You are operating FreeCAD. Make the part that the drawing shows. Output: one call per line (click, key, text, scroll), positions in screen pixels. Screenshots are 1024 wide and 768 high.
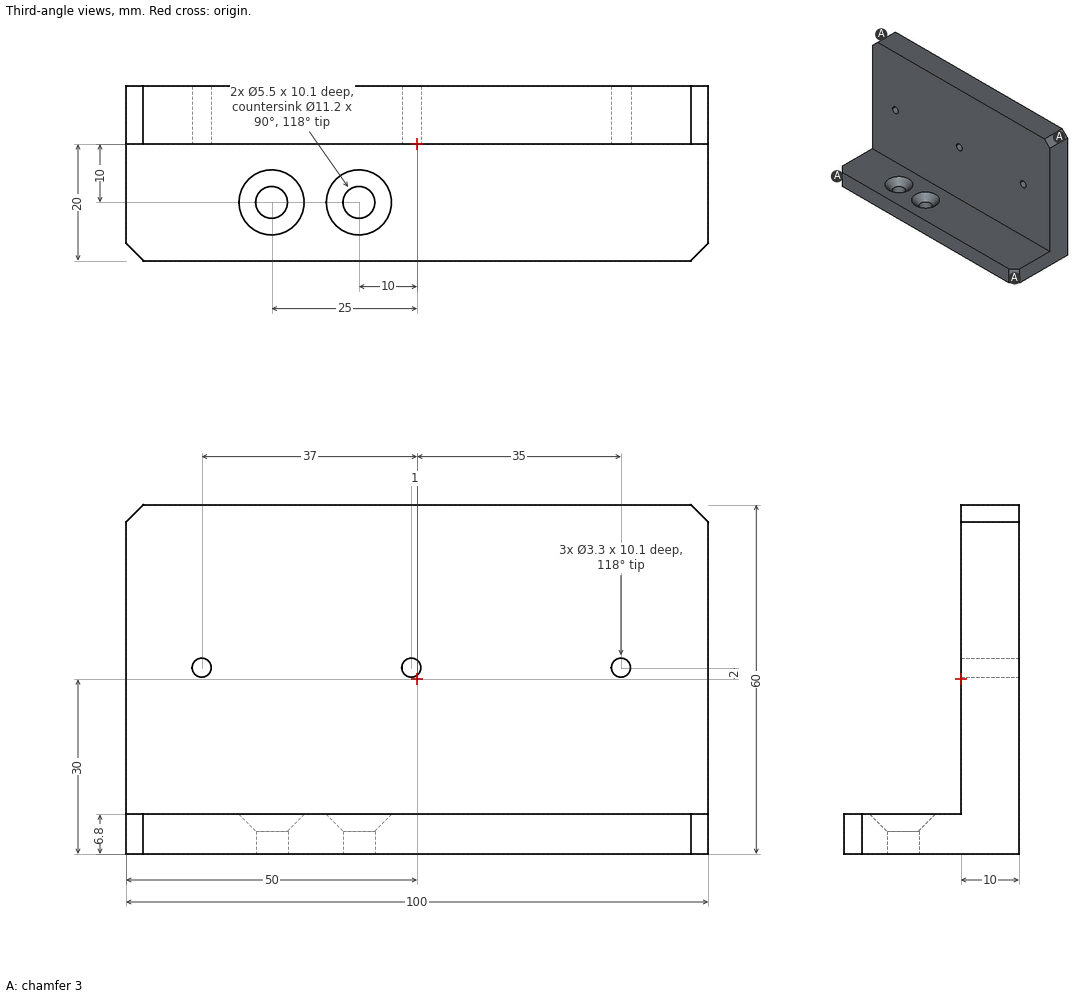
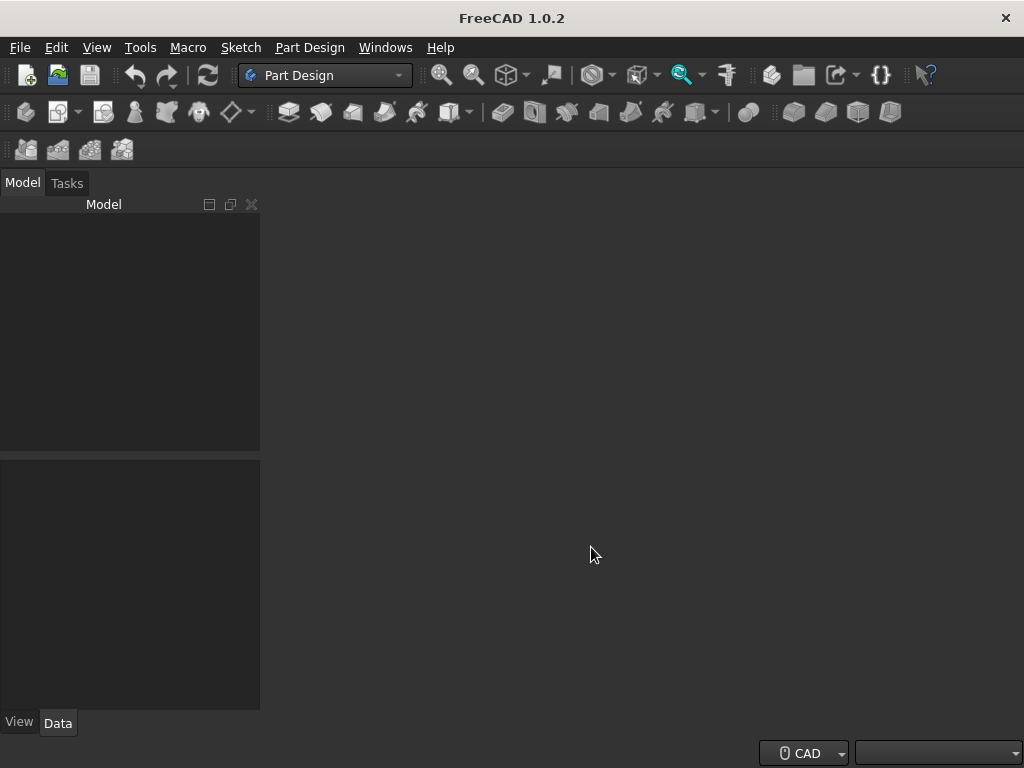
click(26, 76)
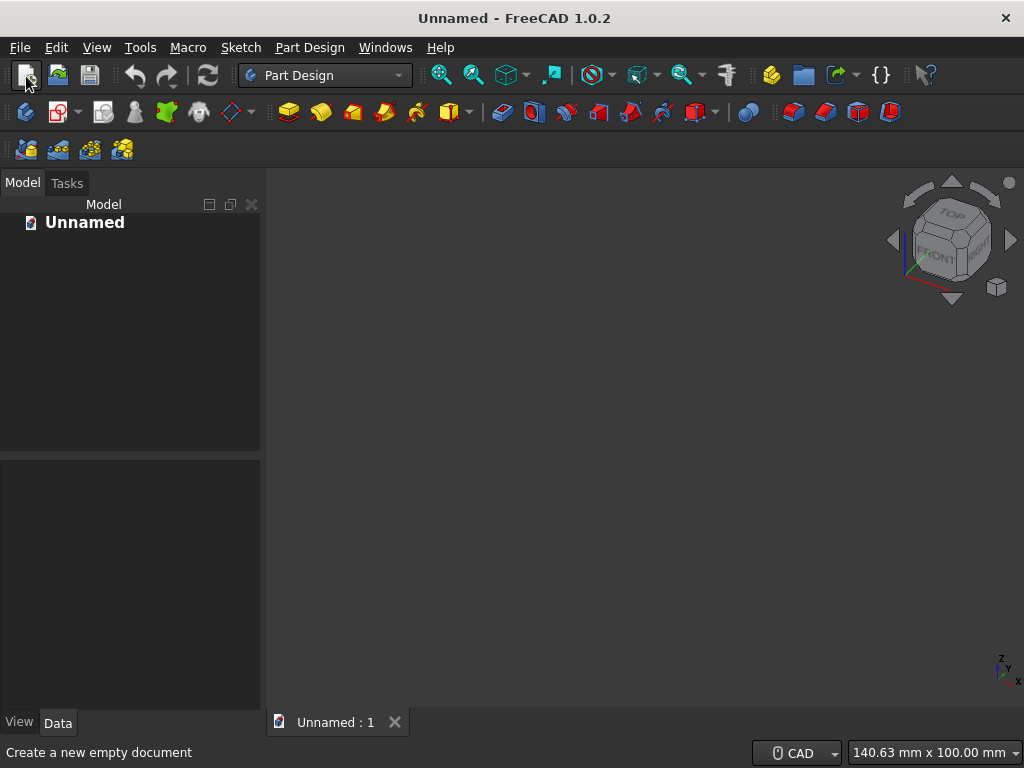
click(58, 112)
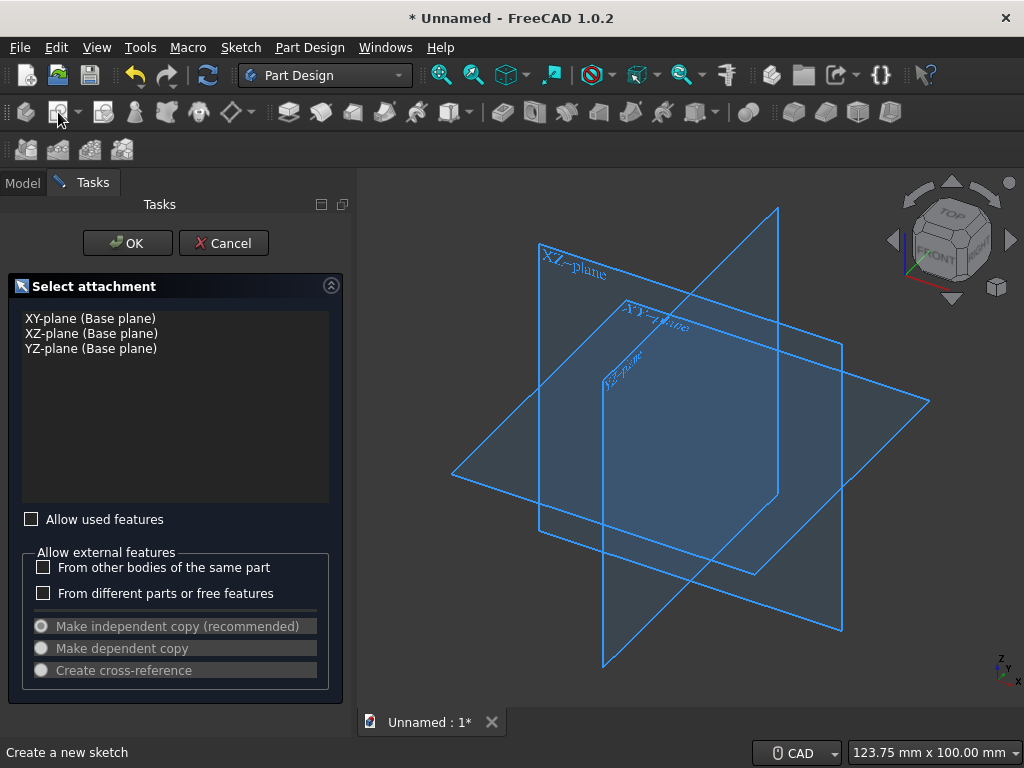
click(82, 334)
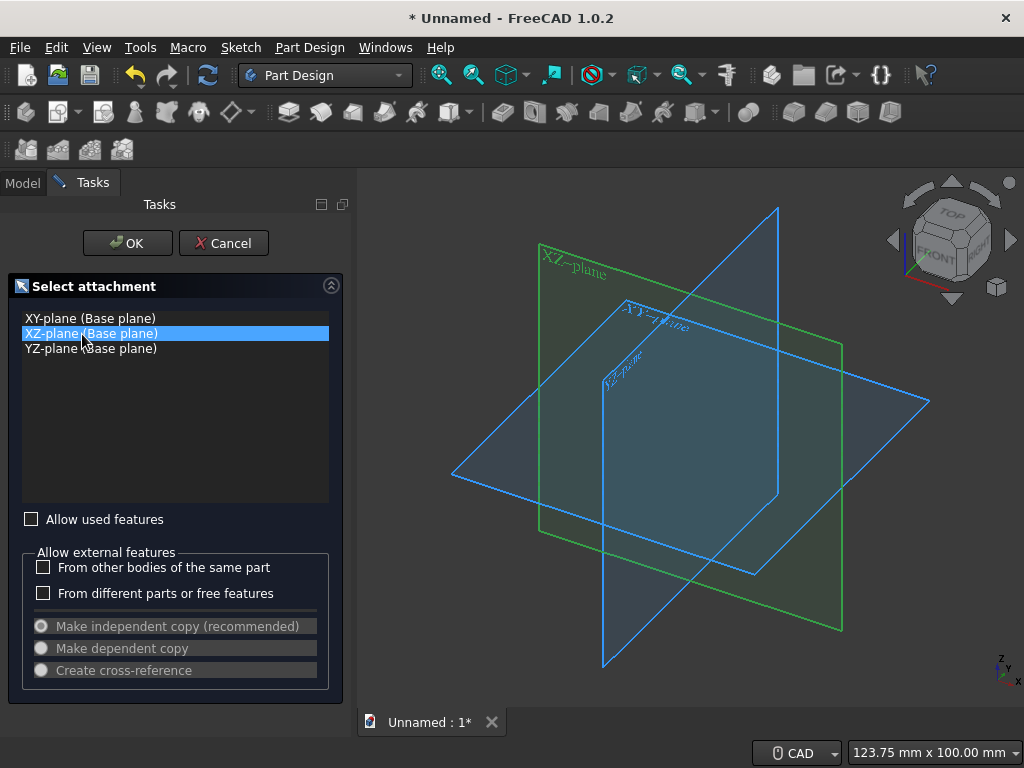
click(128, 243)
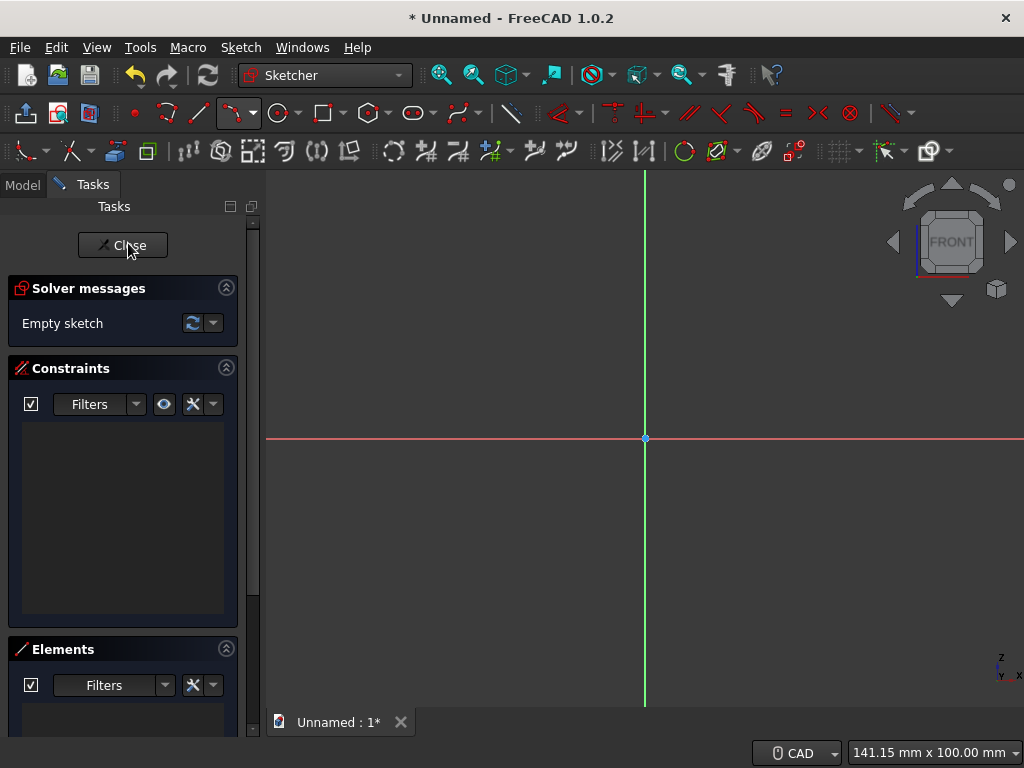
scroll(294, 439, down, 1)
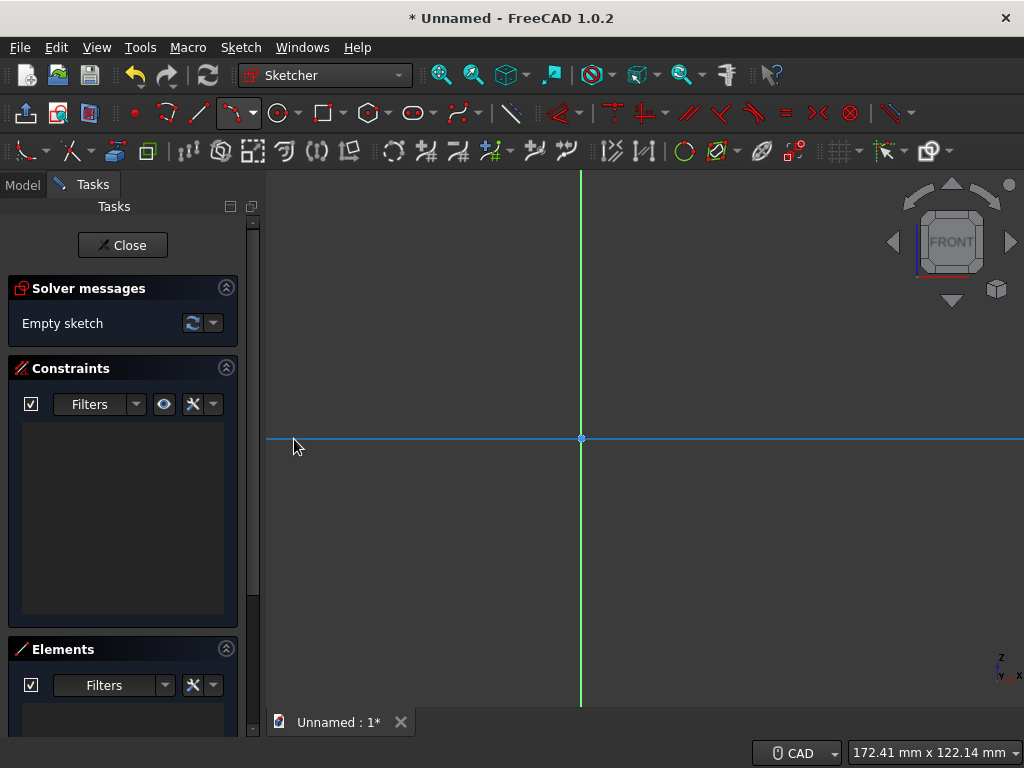
key(g)
key(v)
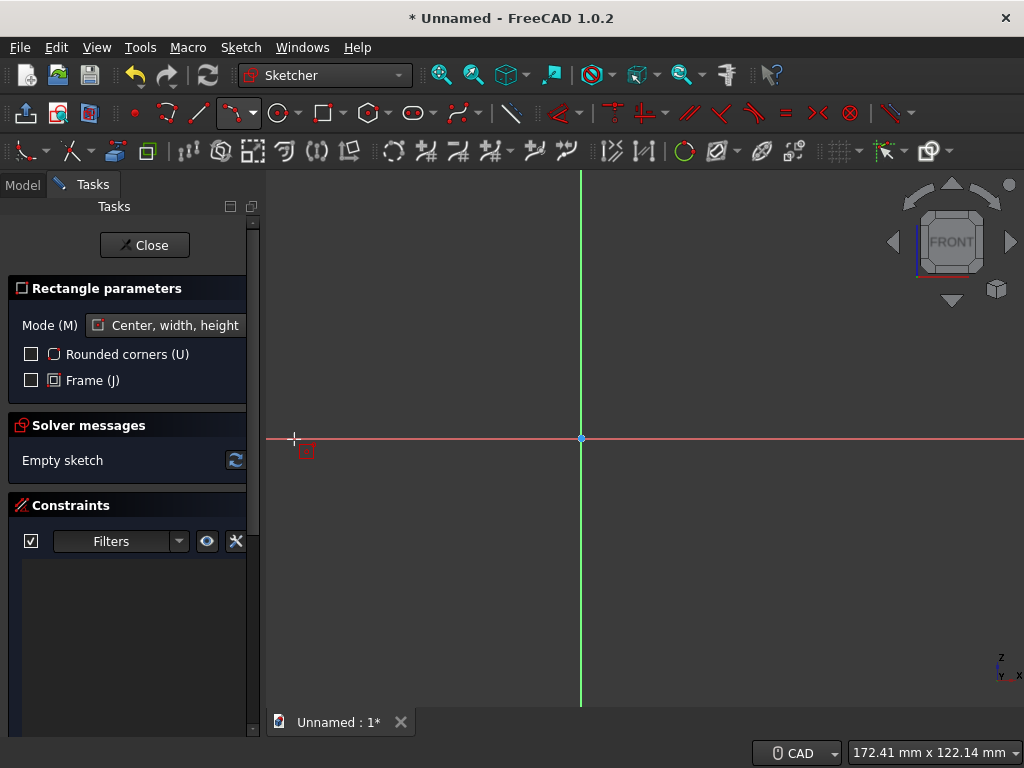
click(581, 439)
click(801, 307)
key(Escape)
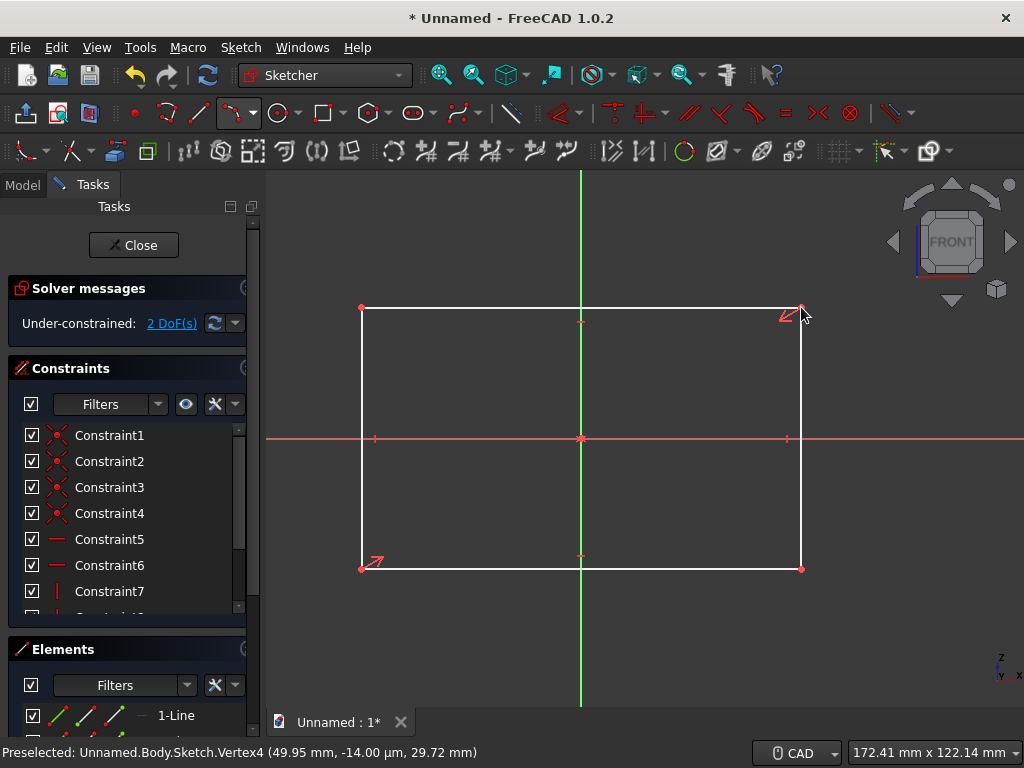
click(558, 114)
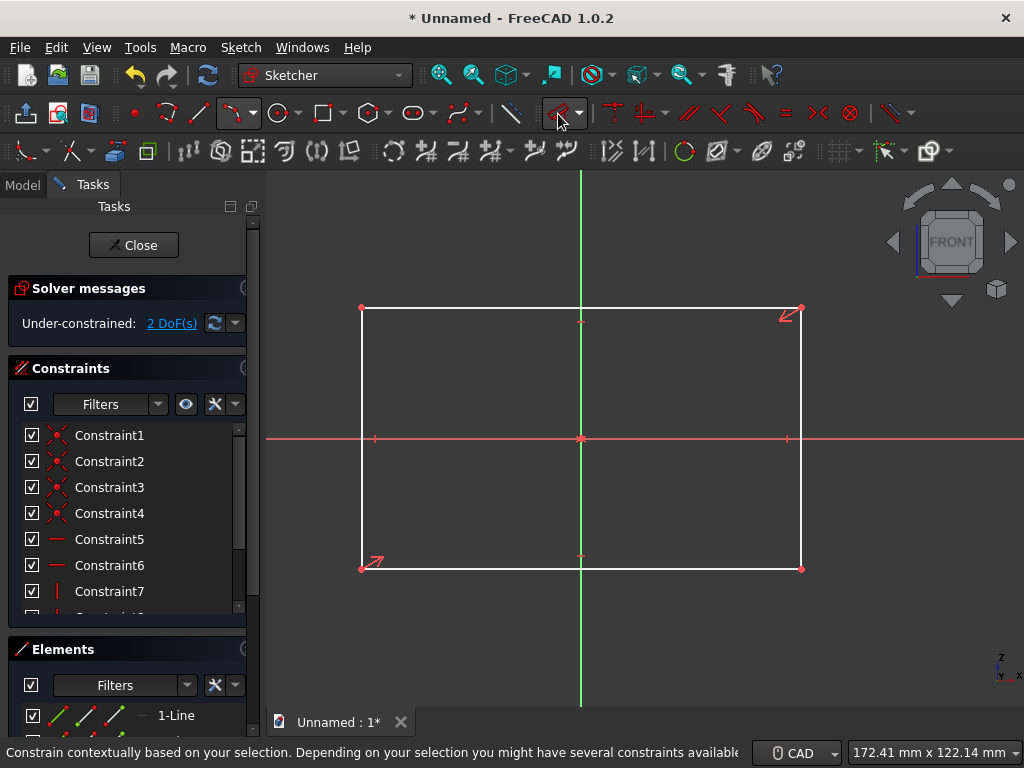
click(801, 491)
click(835, 379)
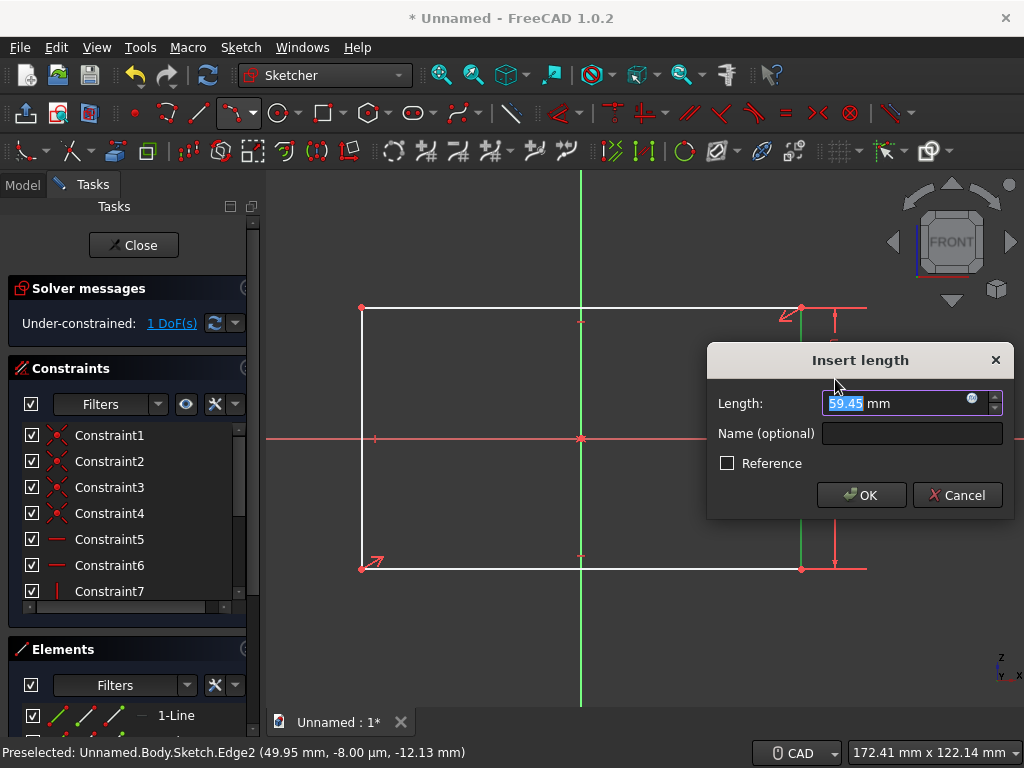
text(60)
key(Return)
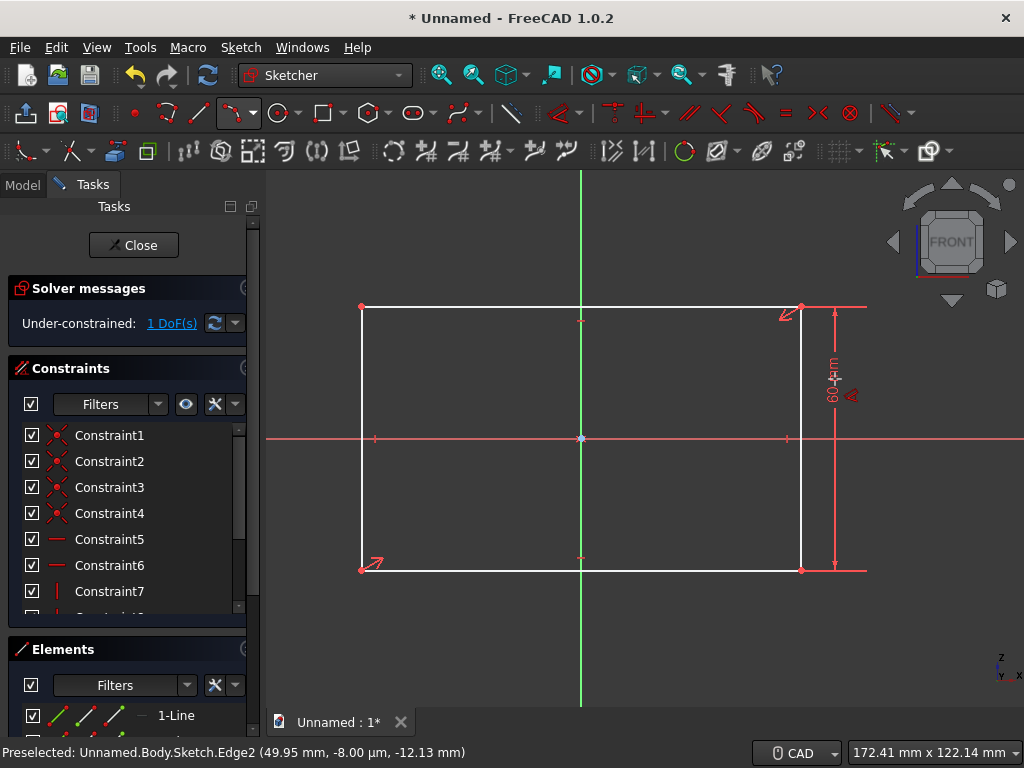
click(494, 571)
click(480, 605)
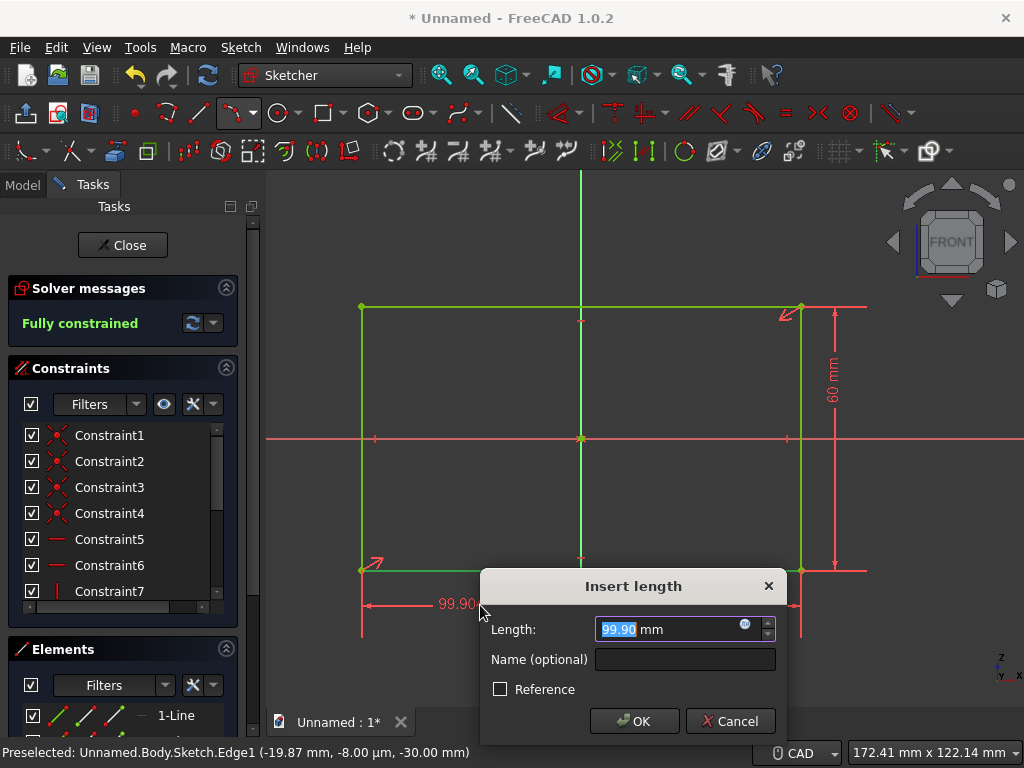
text(100)
key(Return)
key(Escape)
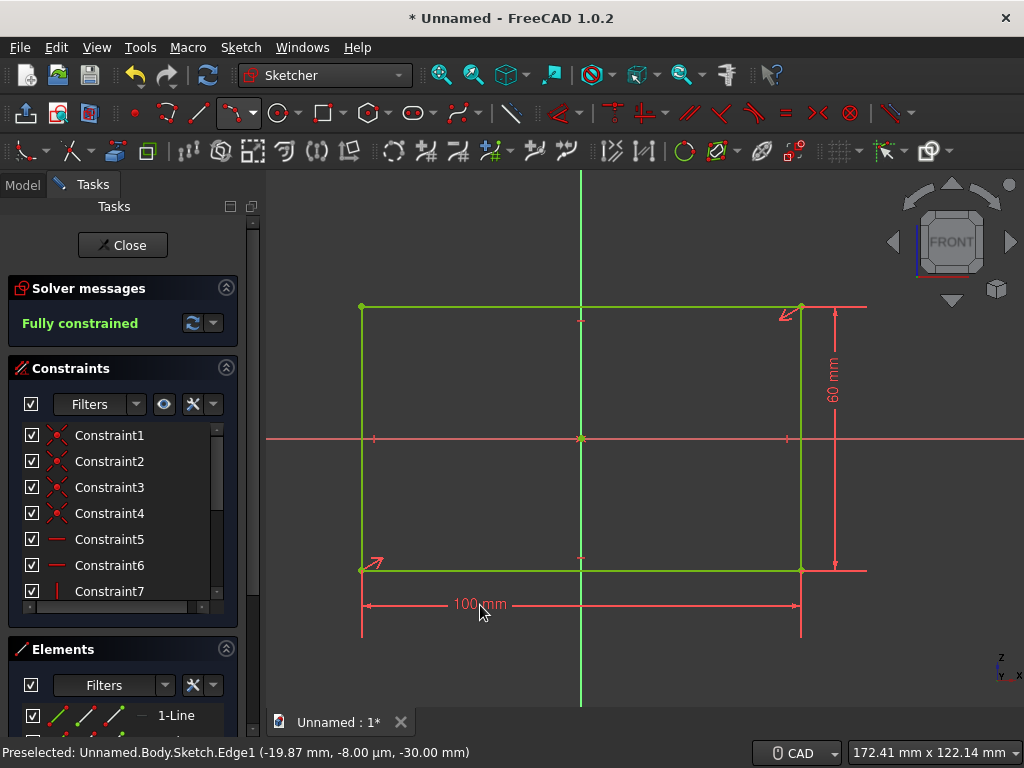
click(123, 245)